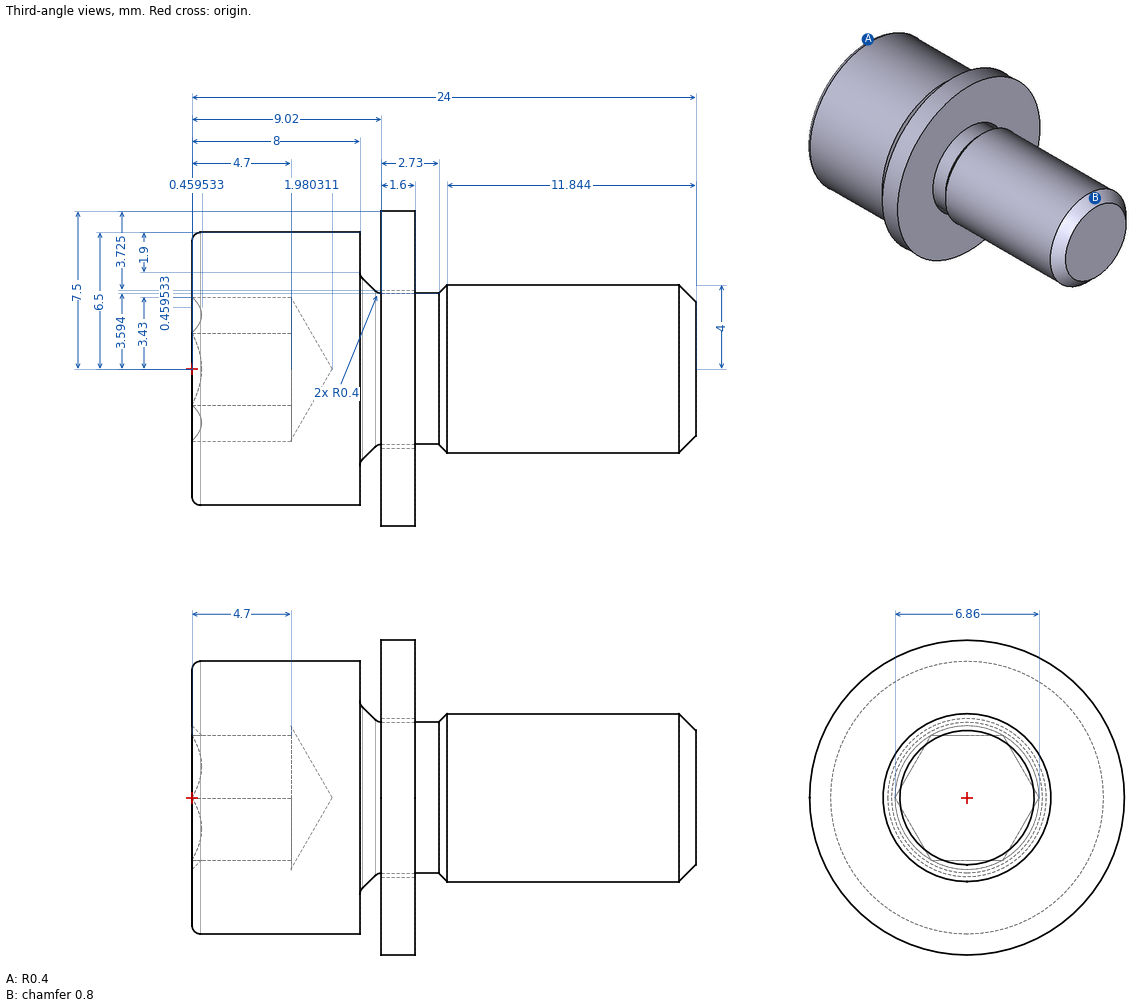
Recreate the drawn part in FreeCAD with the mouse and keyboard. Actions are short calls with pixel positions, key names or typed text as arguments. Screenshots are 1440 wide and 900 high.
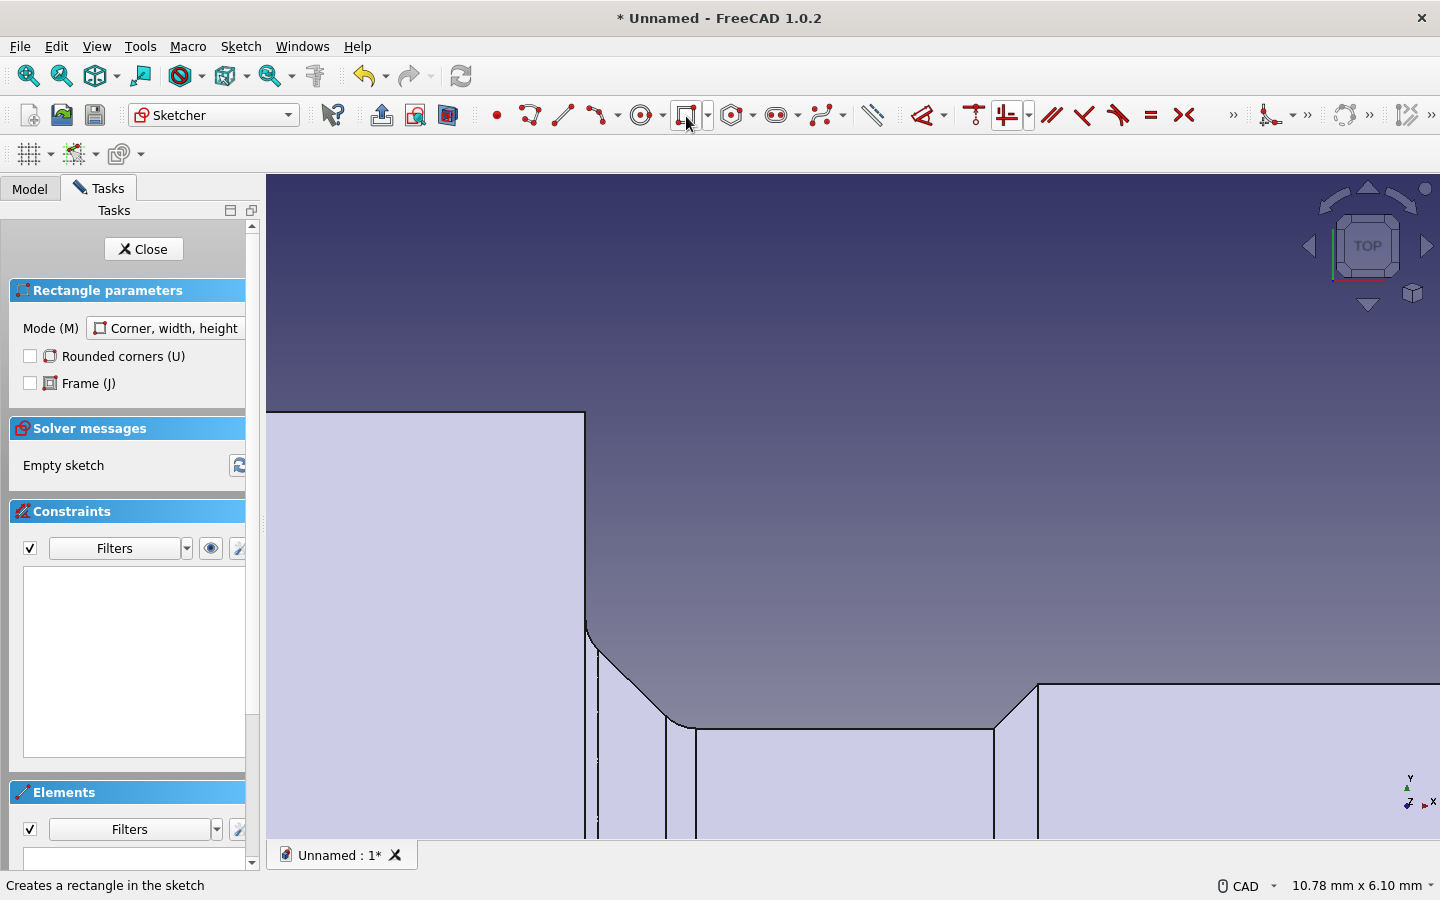
click(696, 303)
click(871, 709)
key(Escape)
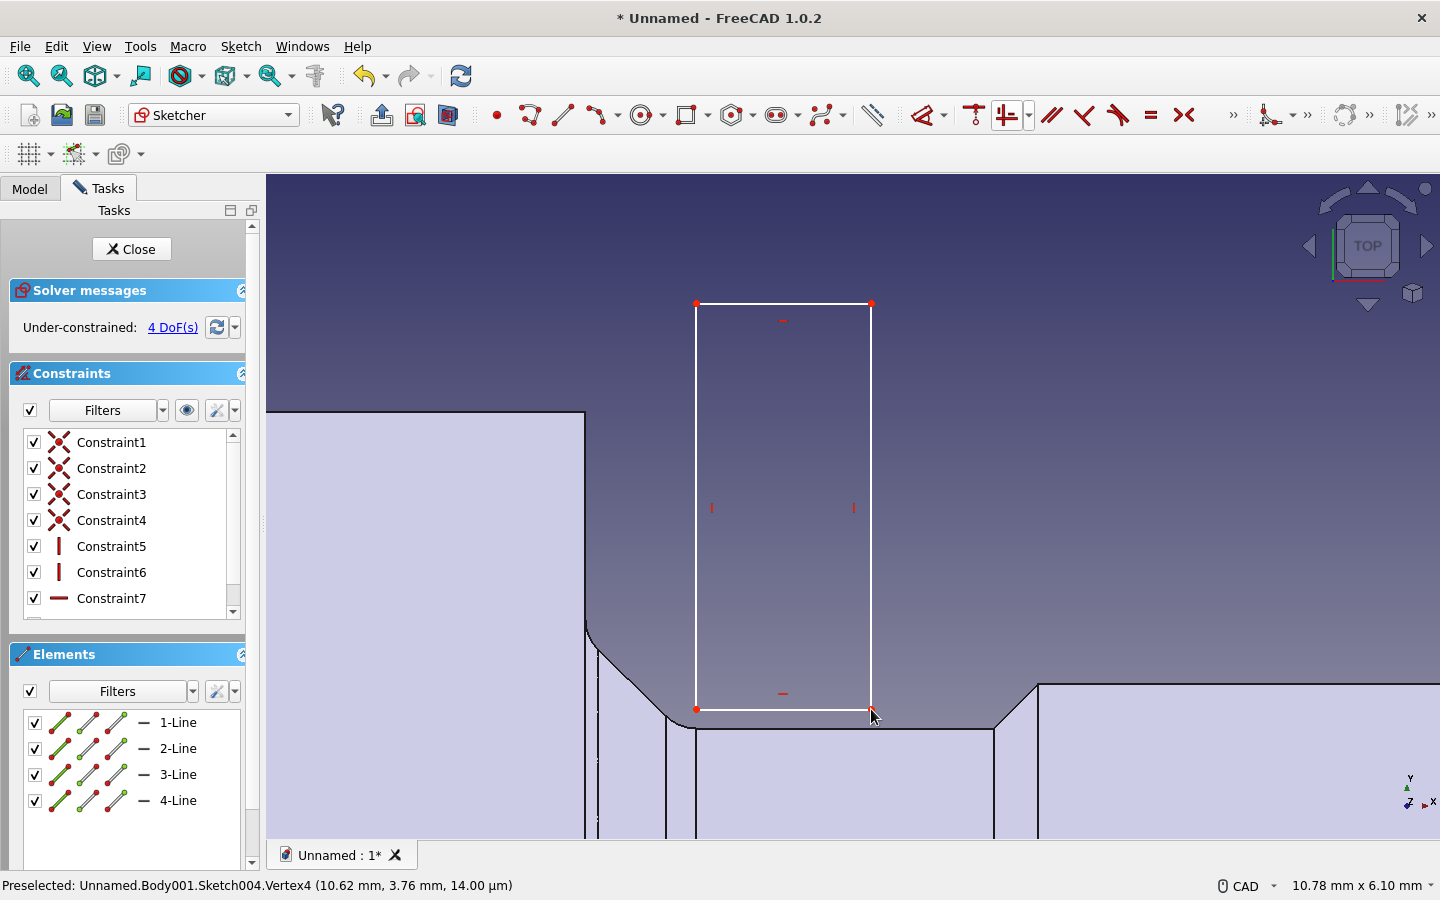
click(922, 116)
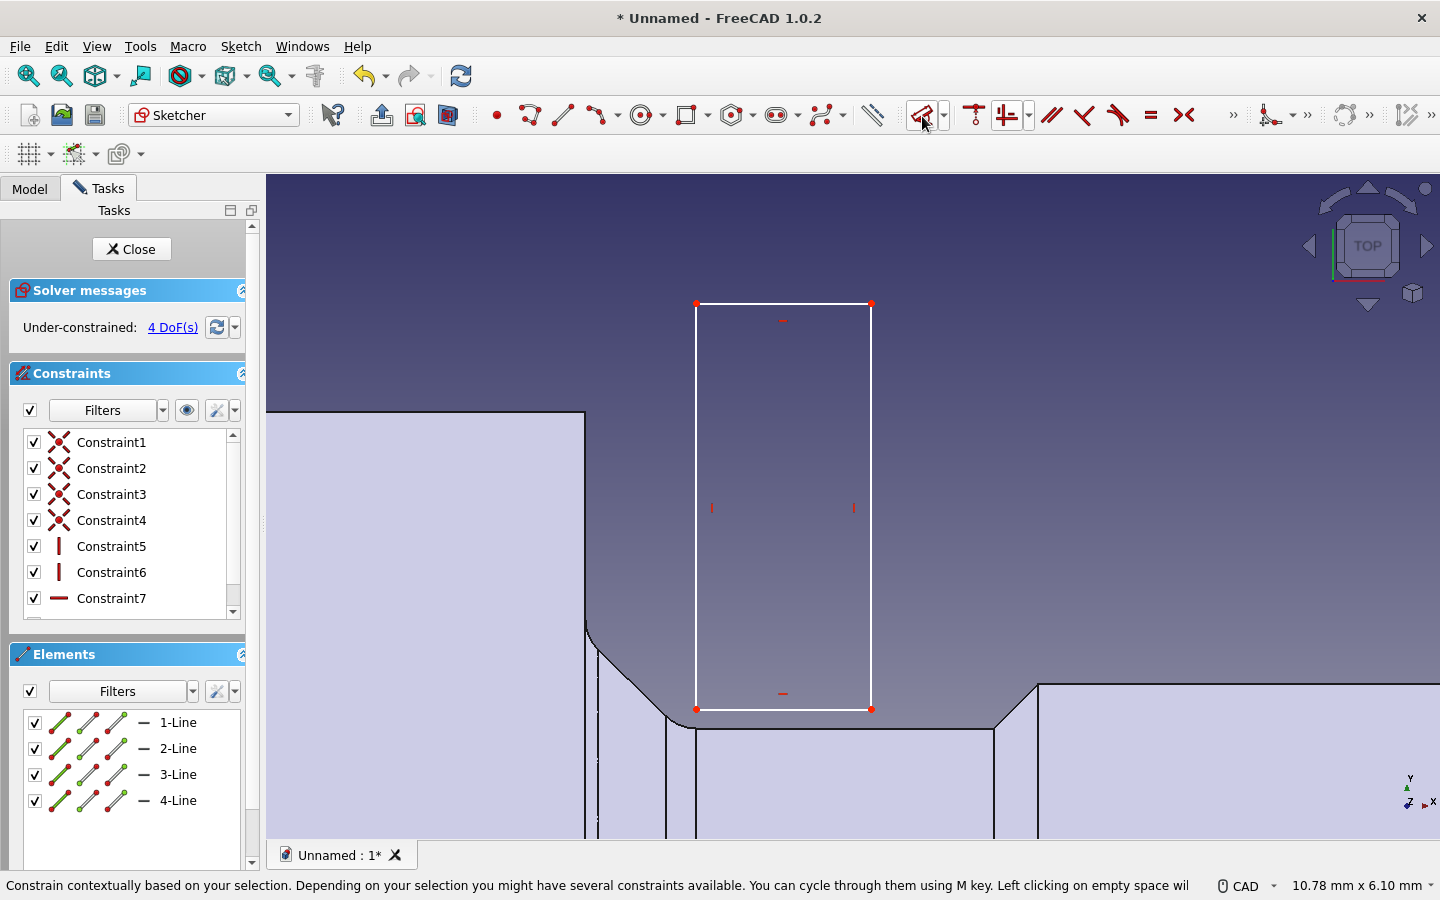
click(748, 710)
click(783, 744)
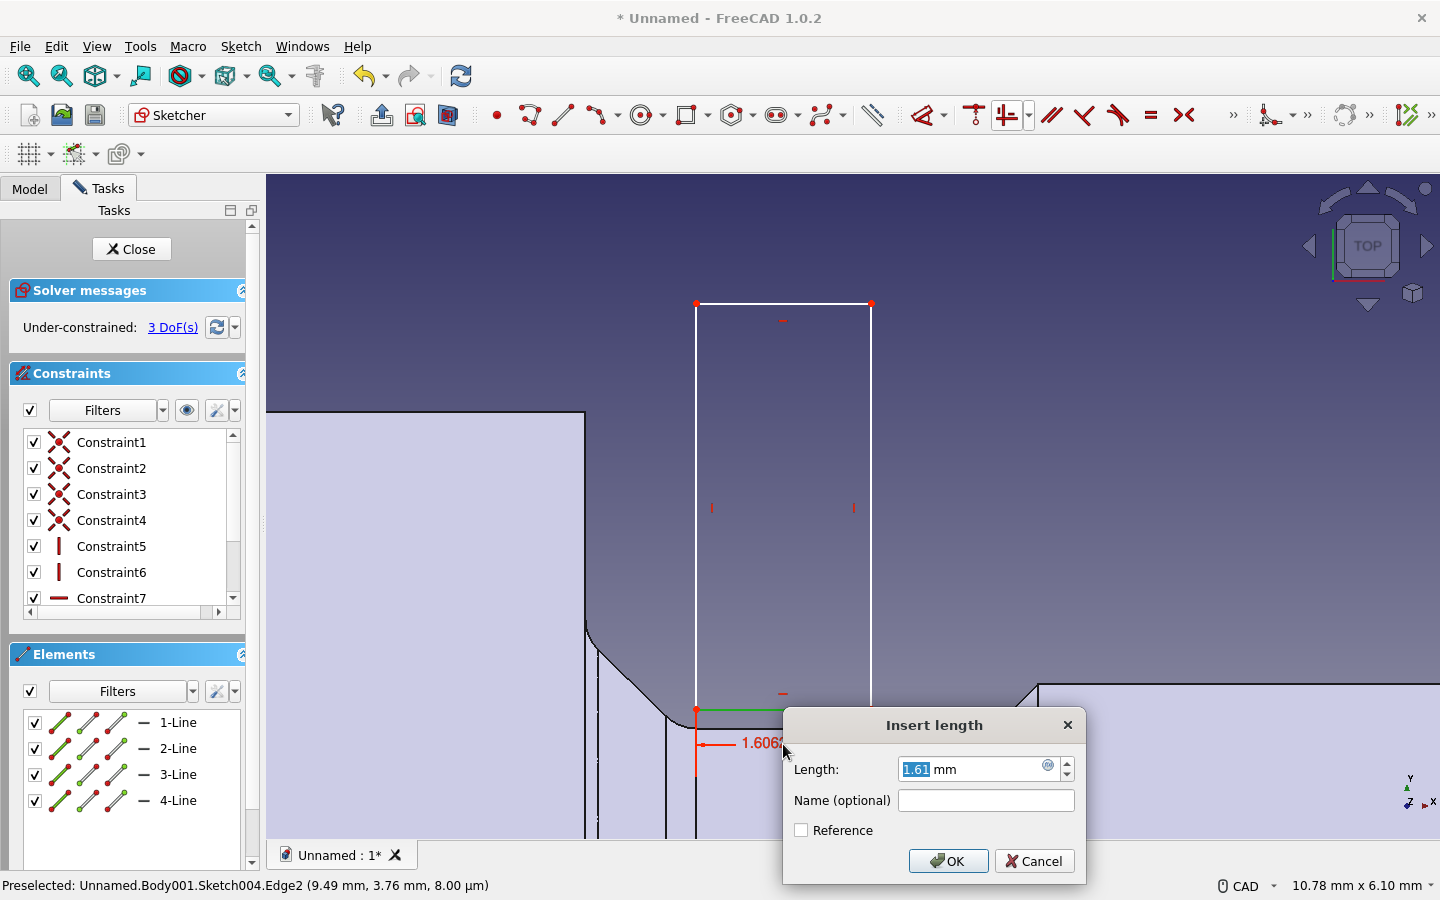
text(1.6)
key(Return)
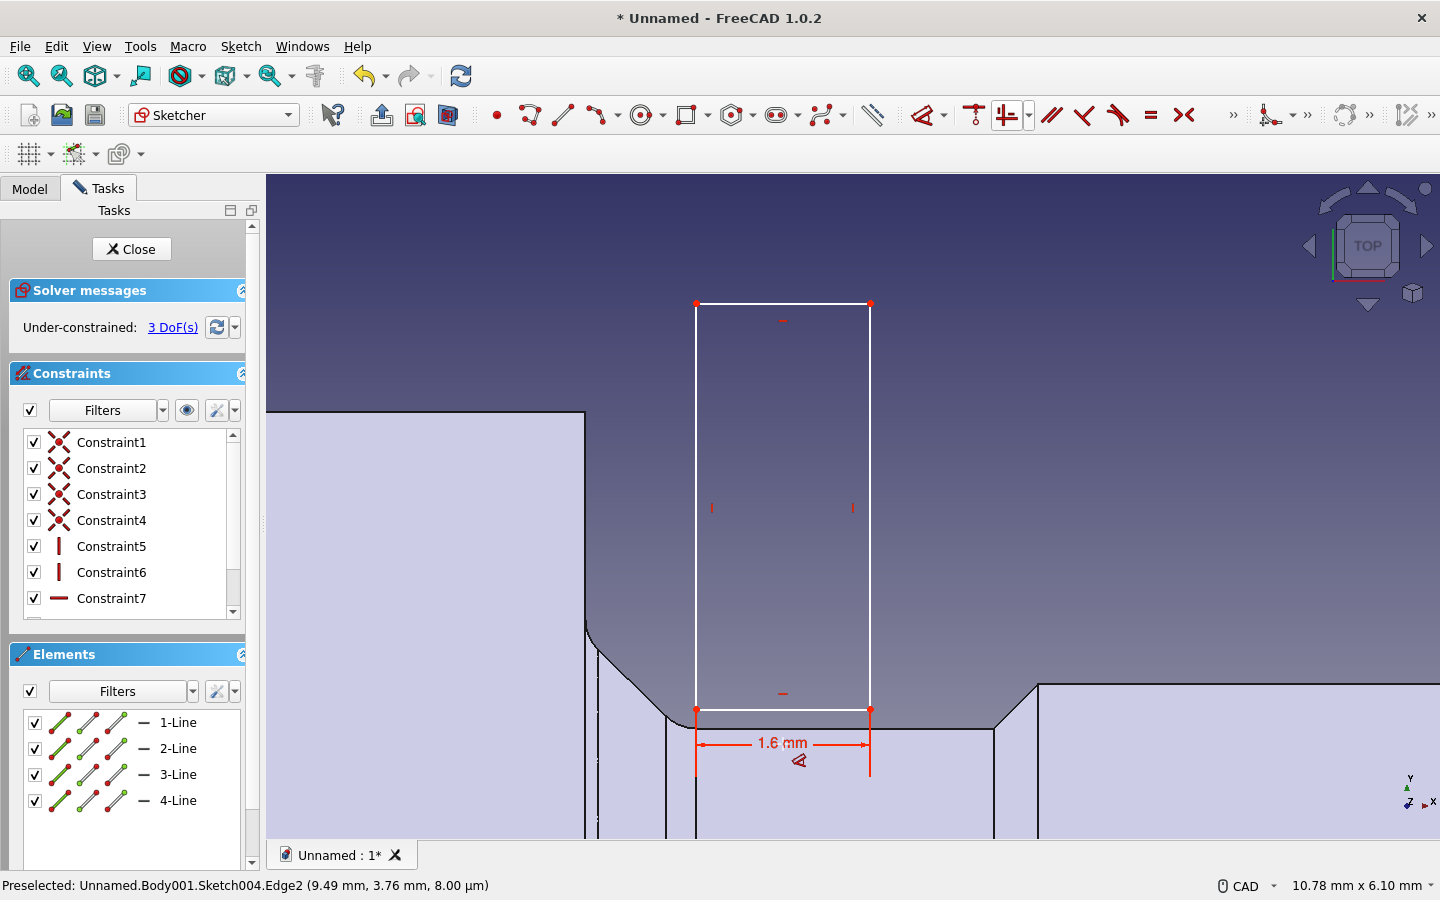
click(696, 304)
click(730, 558)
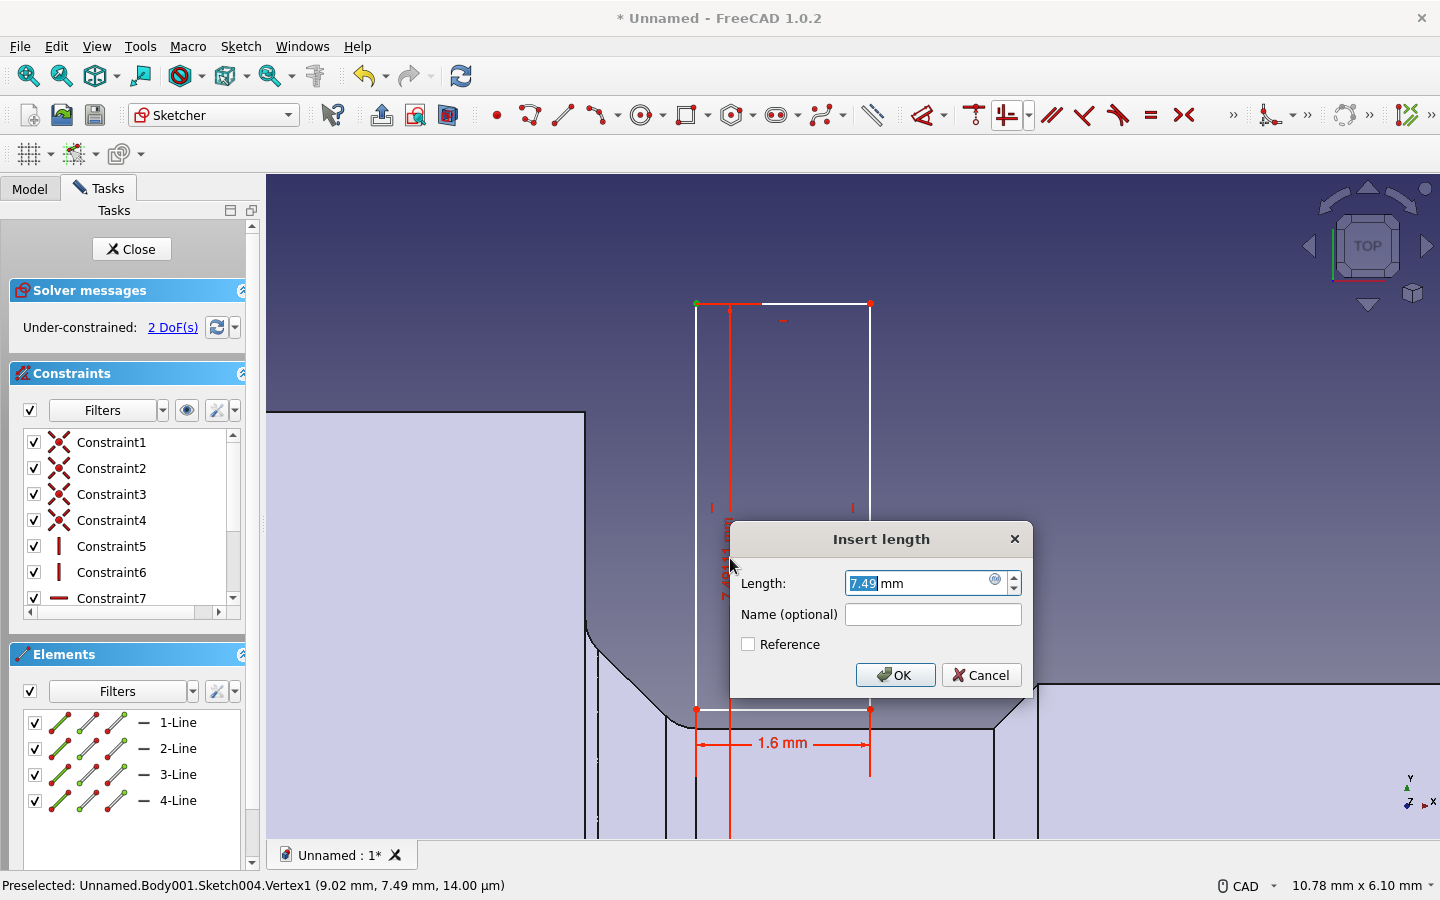
text(7.5)
key(Return)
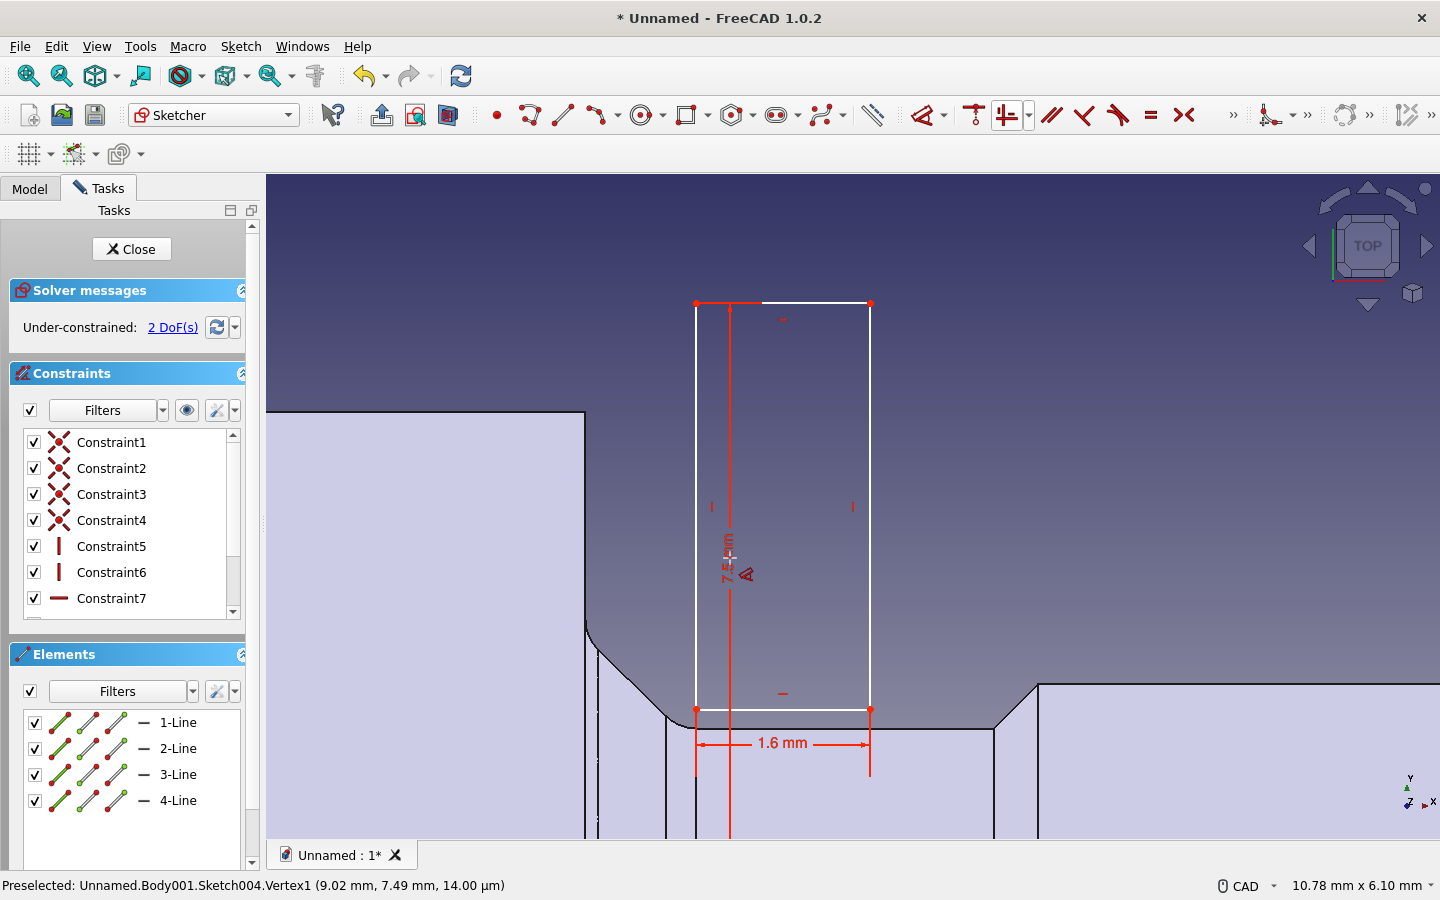
click(696, 425)
click(662, 507)